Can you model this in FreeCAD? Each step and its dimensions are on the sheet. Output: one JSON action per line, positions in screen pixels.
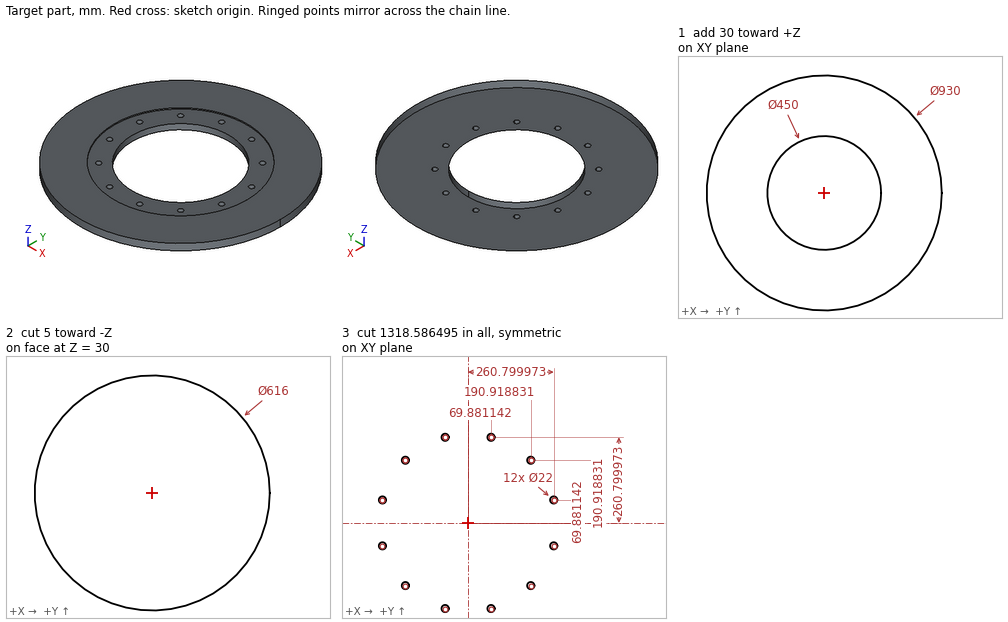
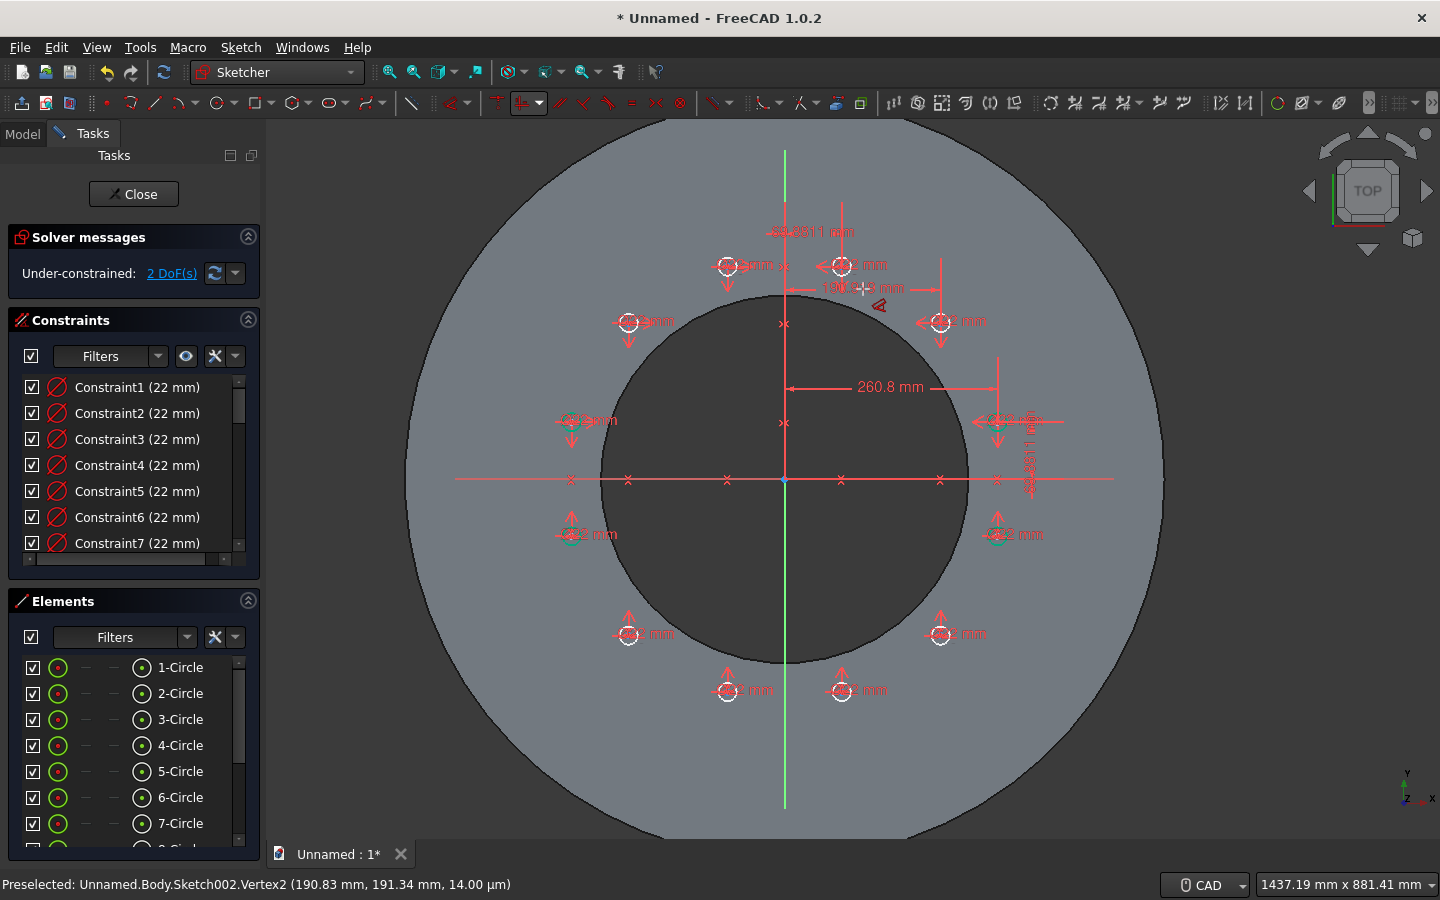
{"action": "left_click", "coordinate": [941, 323]}
{"action": "left_click", "coordinate": [975, 401]}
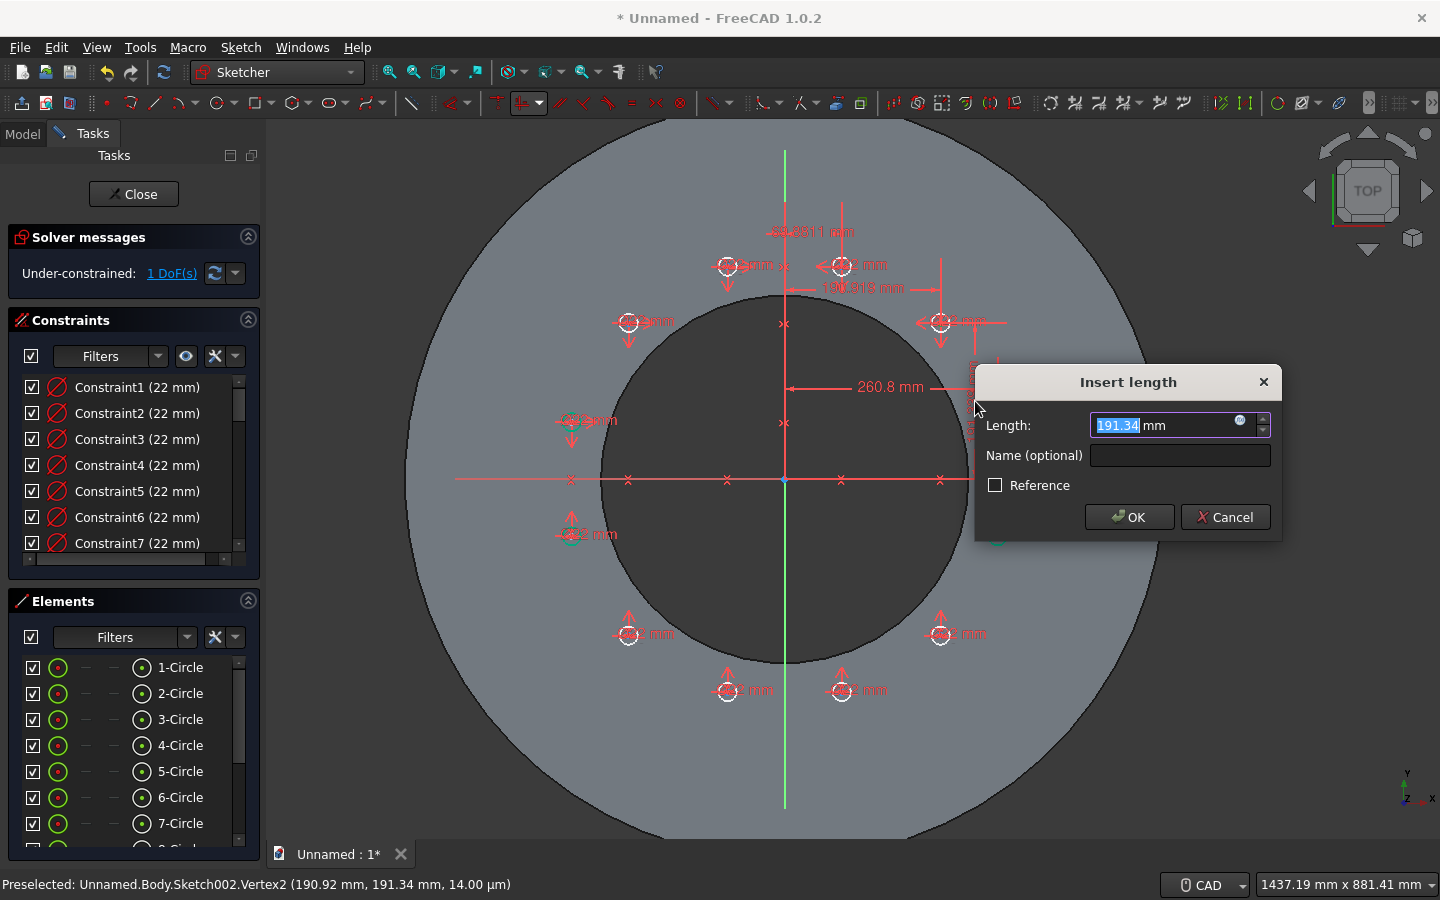
{"action": "type", "text": "190.918831"}
{"action": "key", "text": "Return"}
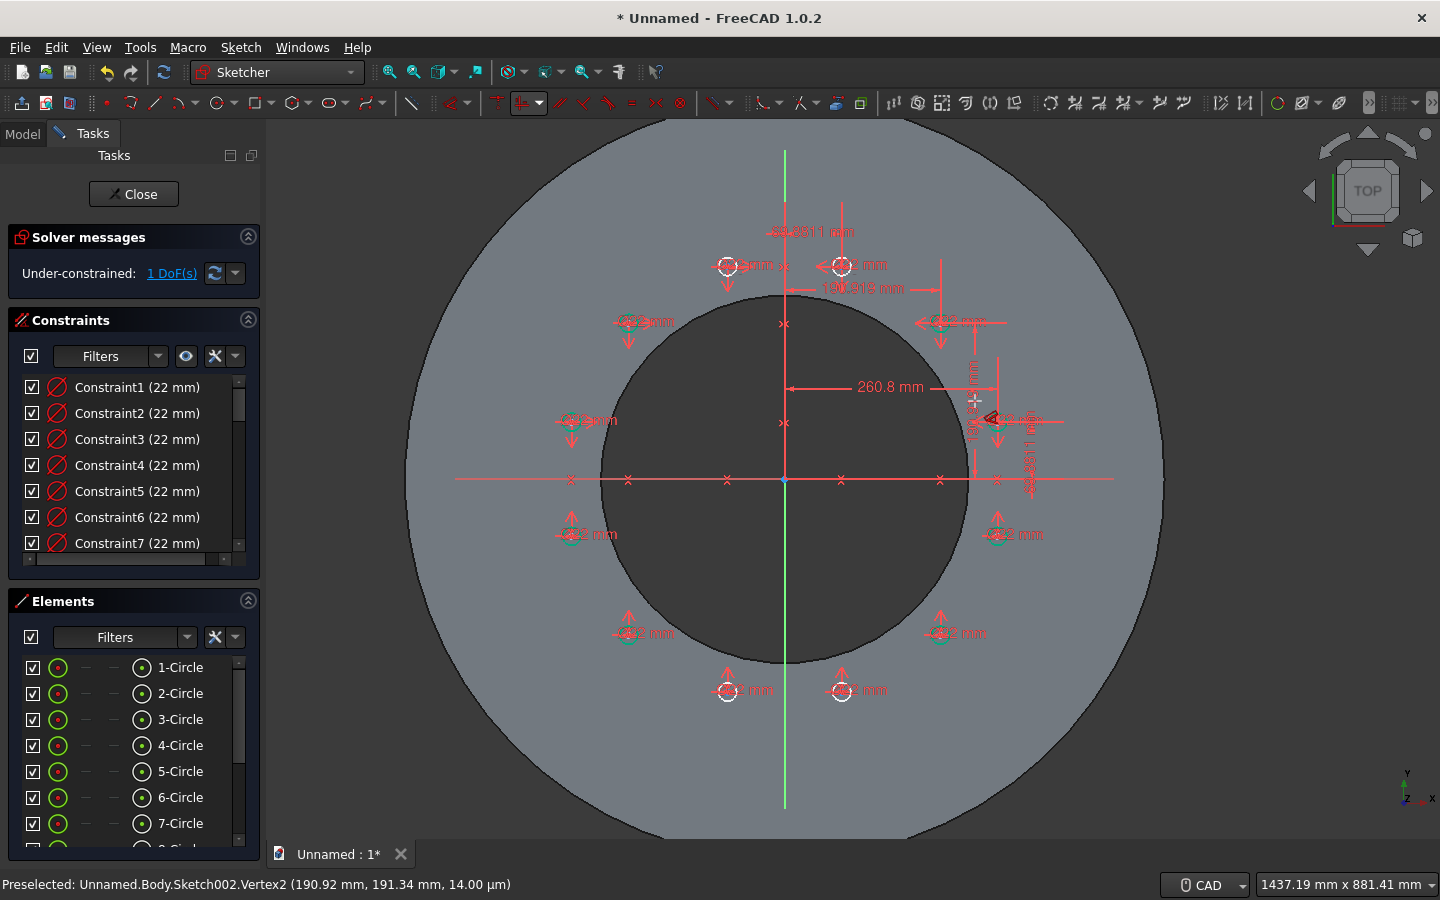
{"action": "left_click", "coordinate": [842, 267]}
{"action": "left_click", "coordinate": [876, 324]}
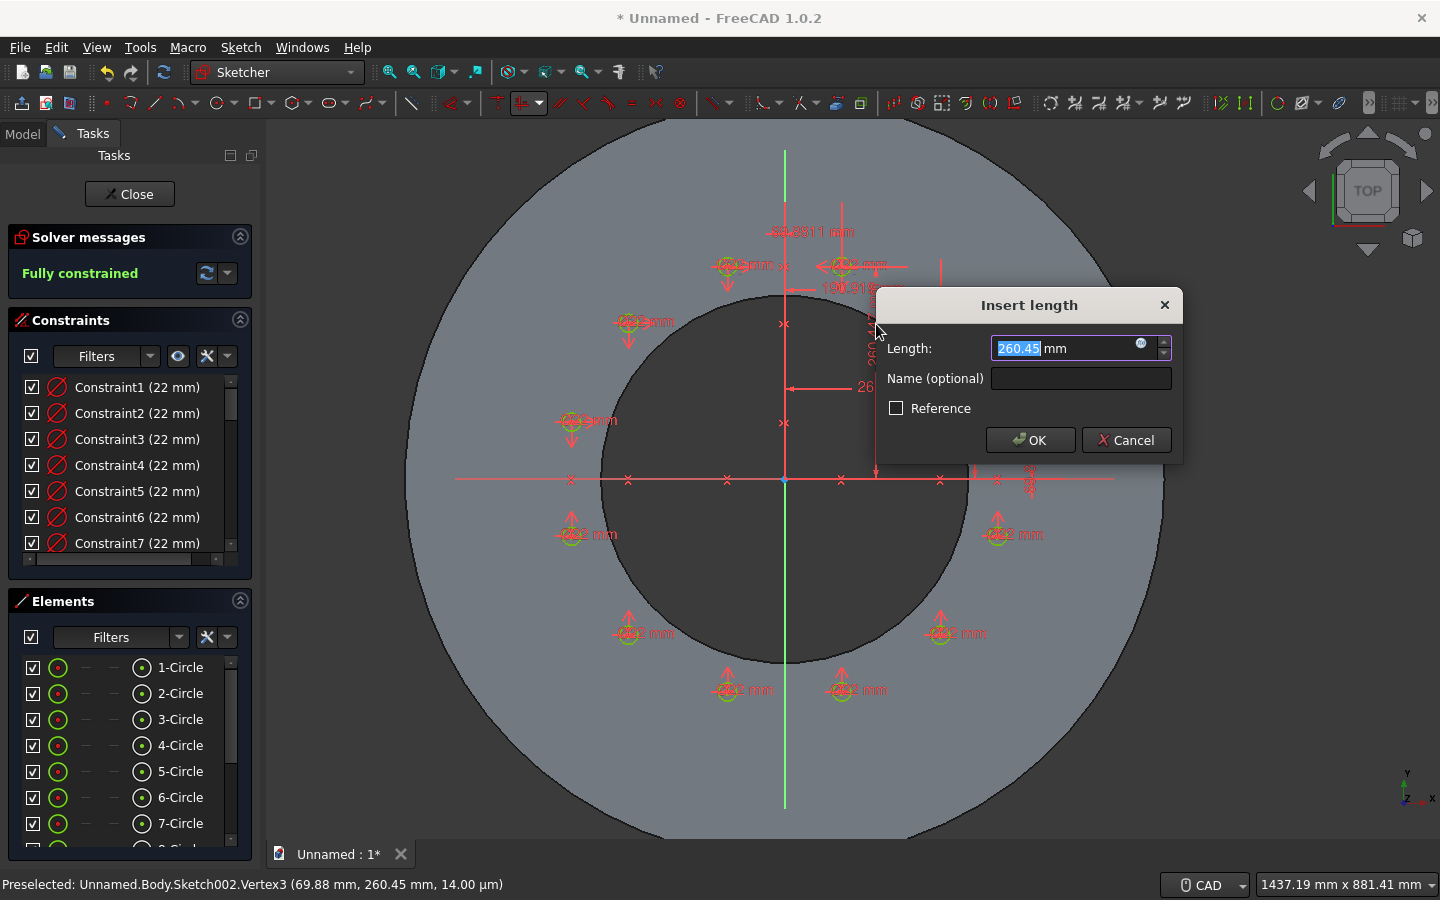
{"action": "type", "text": "260.799973"}
{"action": "key", "text": "Return"}
{"action": "key", "text": "Escape"}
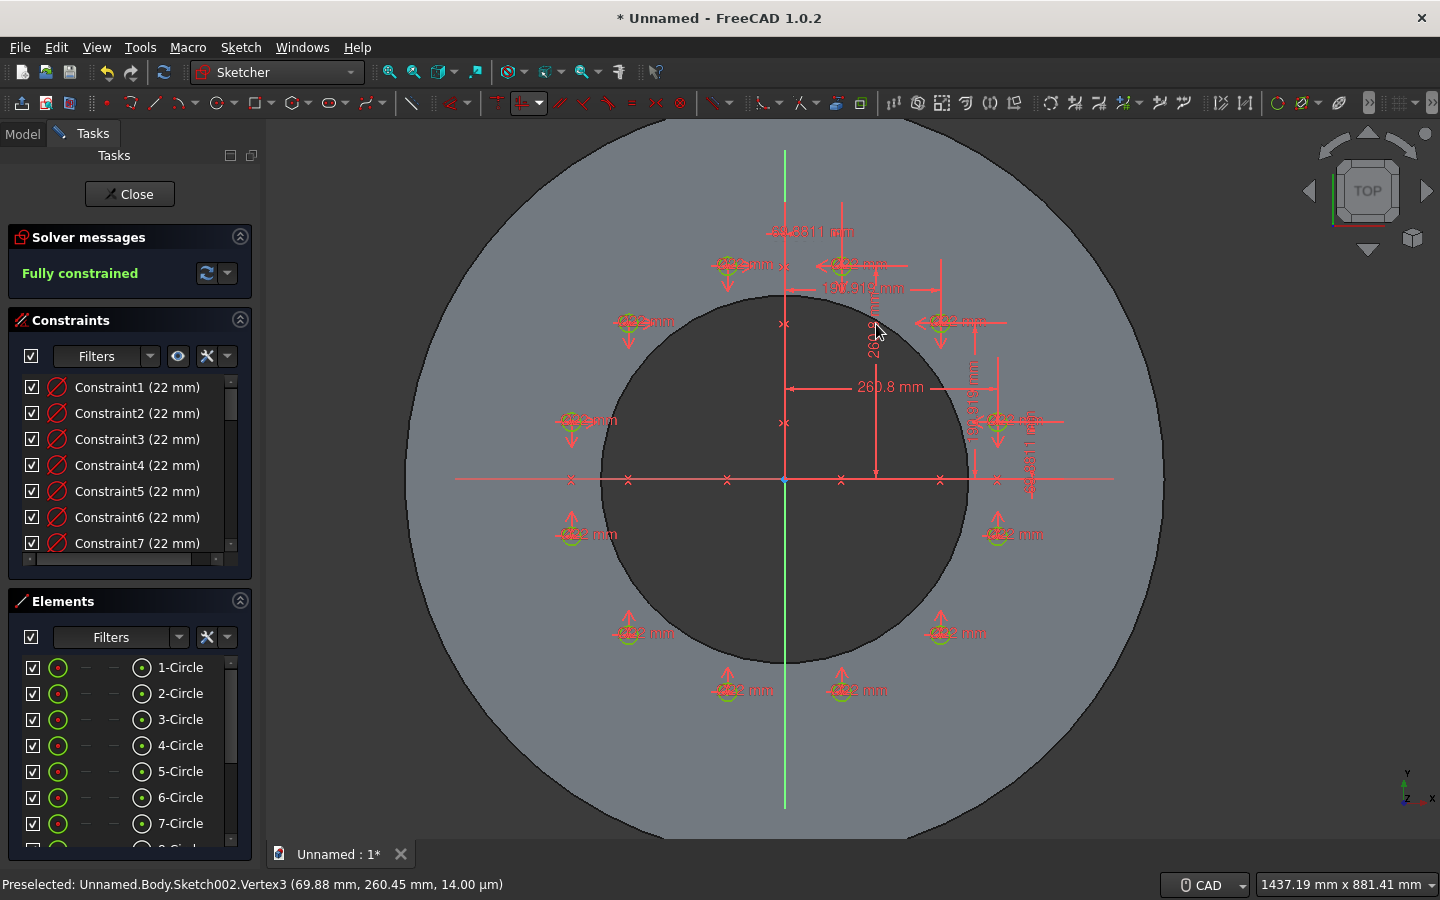
{"action": "left_click", "coordinate": [130, 194]}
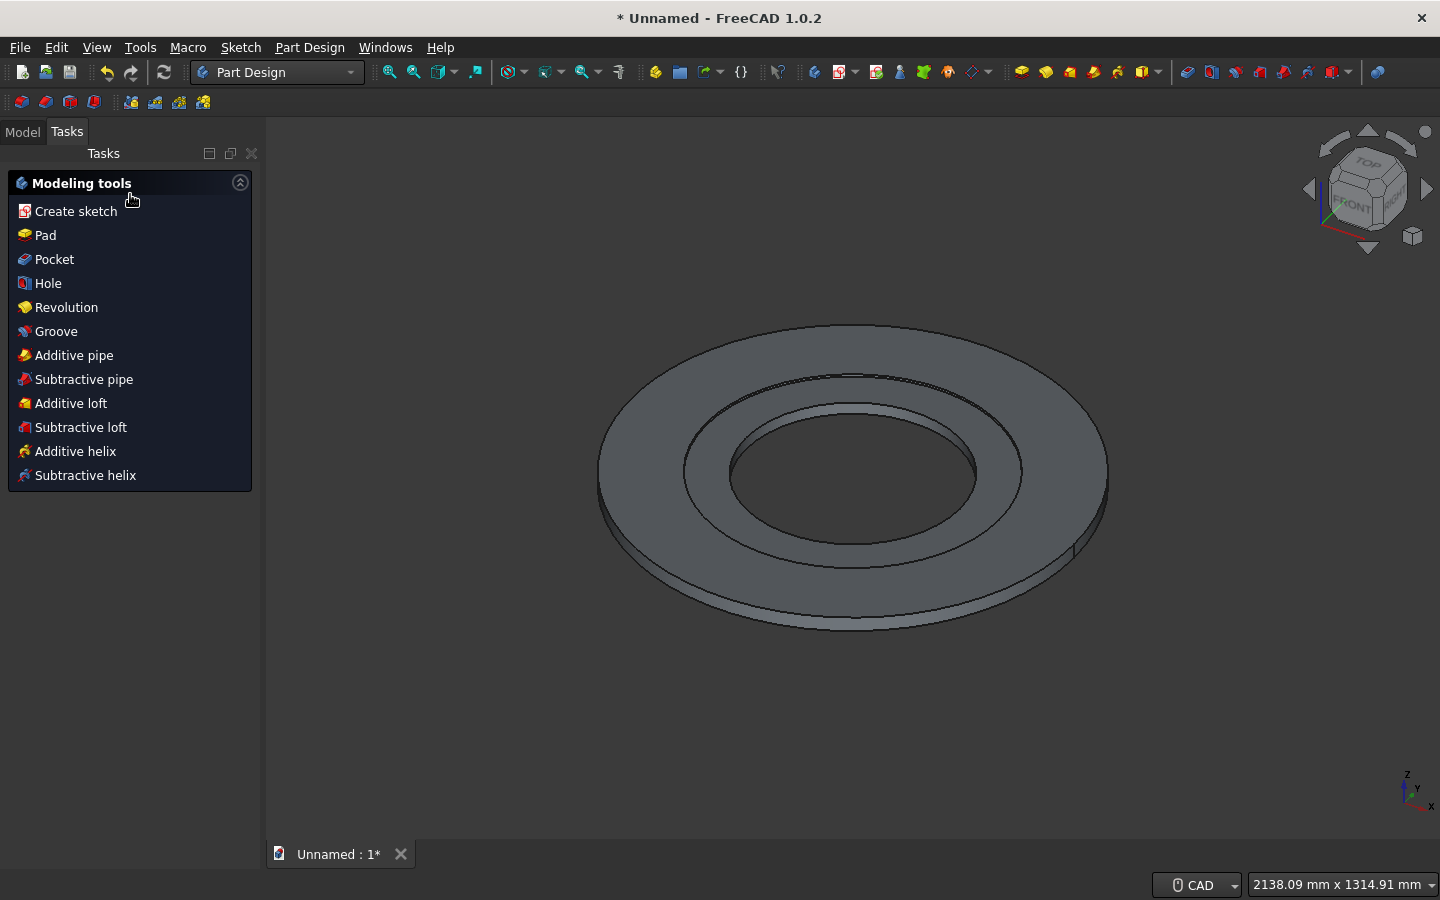
{"action": "left_click", "coordinate": [1188, 72]}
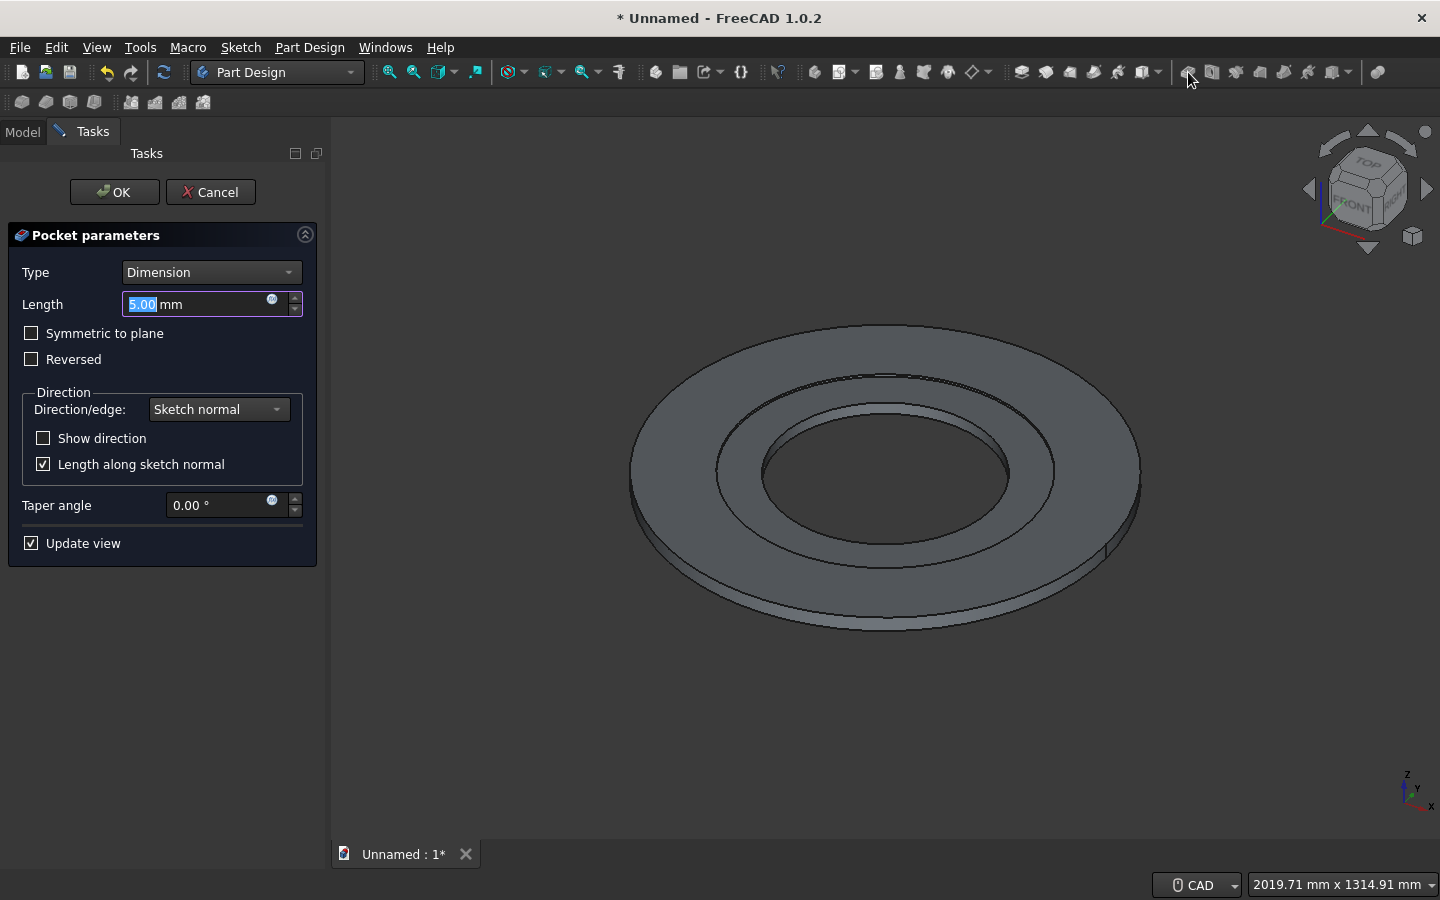
{"action": "type", "text": "1318.586495"}
{"action": "key", "text": "Tab"}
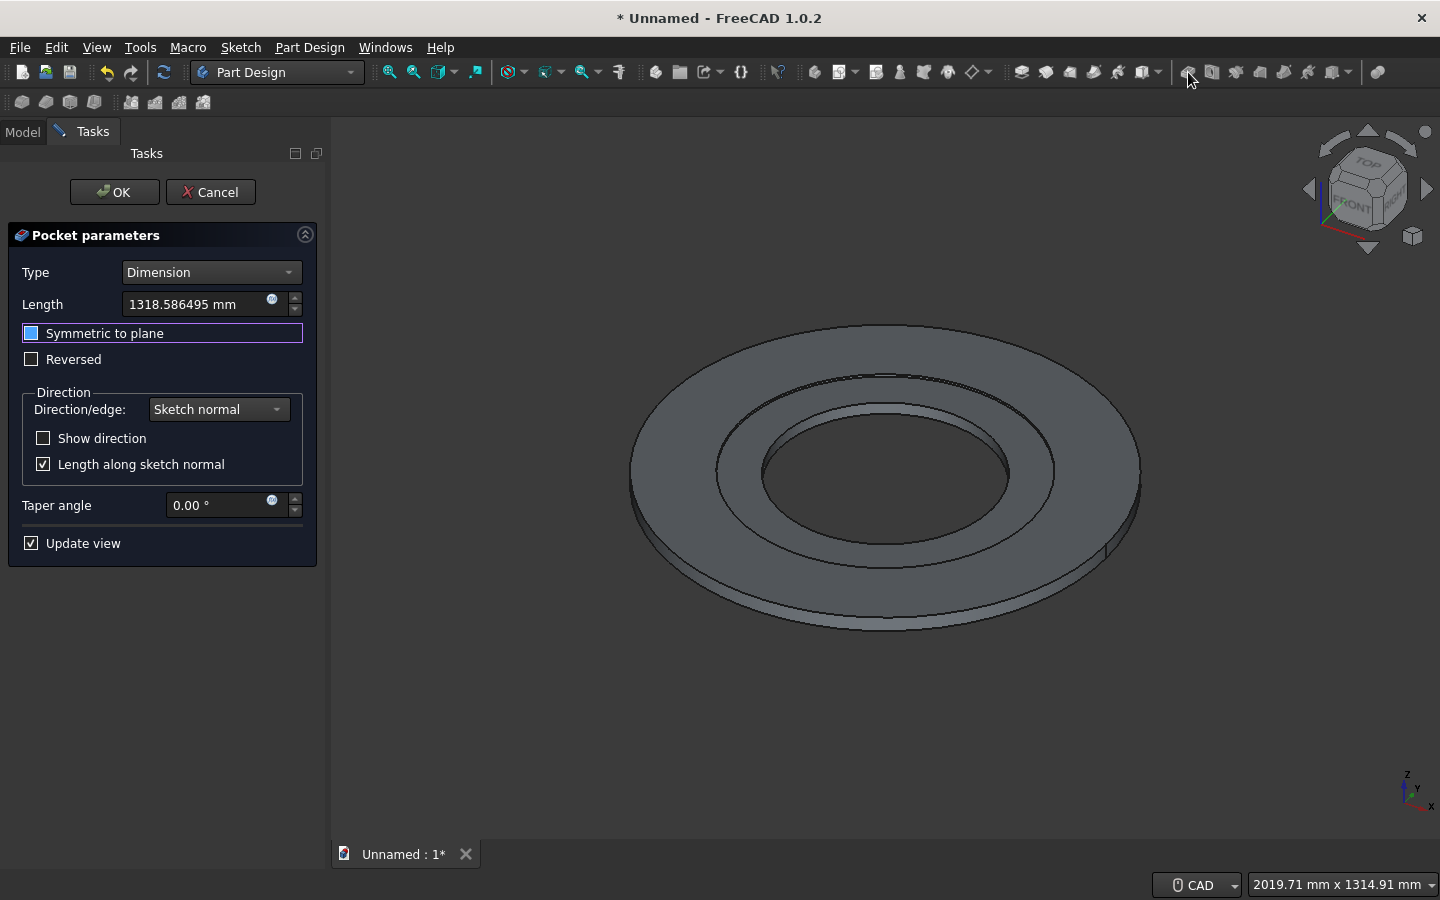
{"action": "left_click", "coordinate": [30, 333]}